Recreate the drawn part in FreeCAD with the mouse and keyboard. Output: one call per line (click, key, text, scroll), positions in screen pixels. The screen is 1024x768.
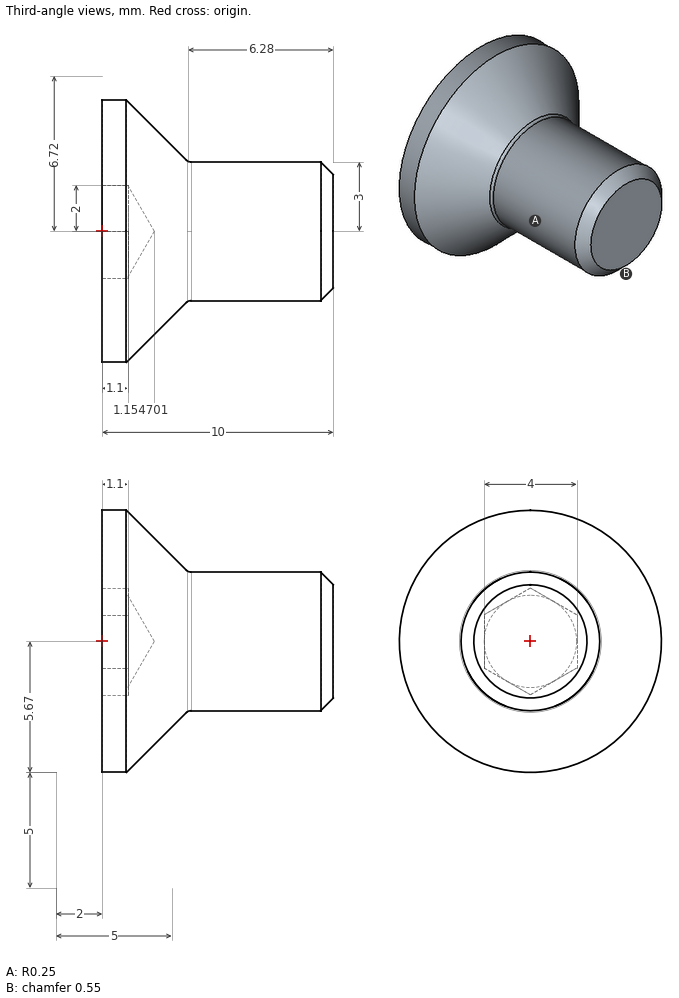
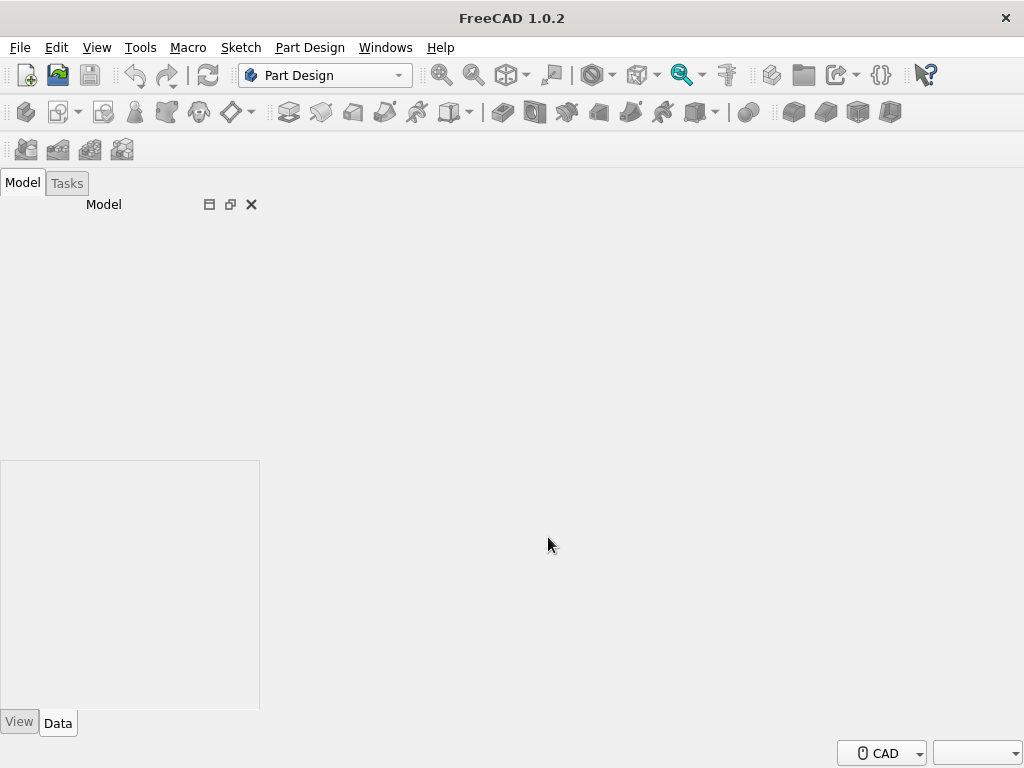
key(ctrl+n)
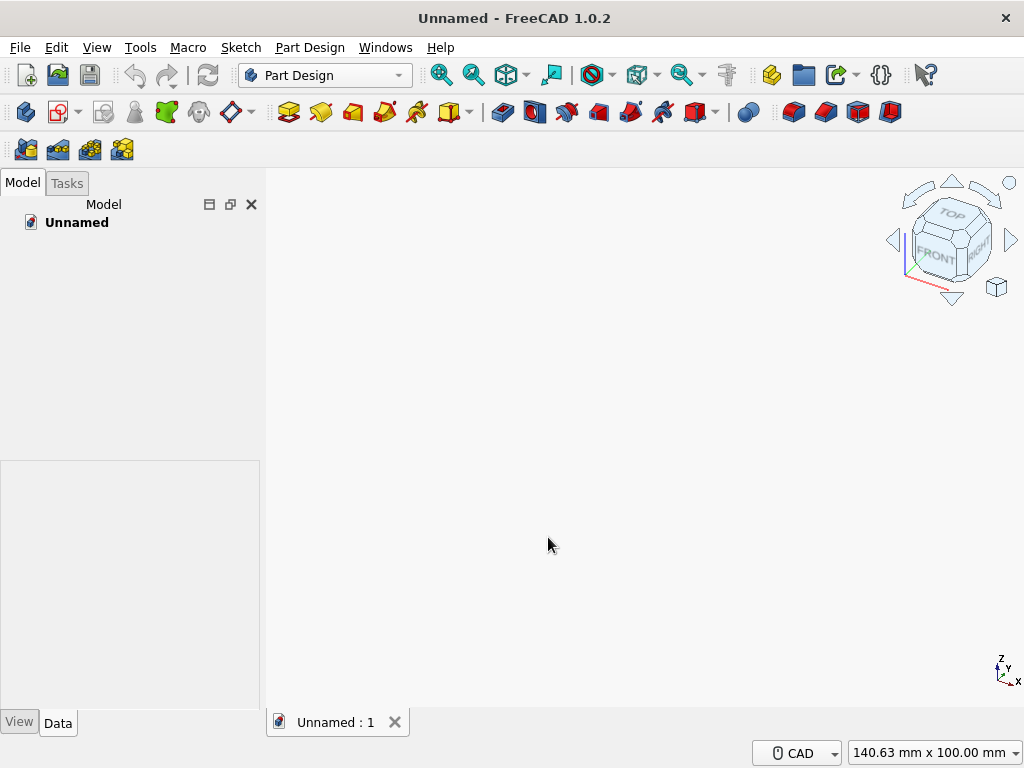
click(58, 112)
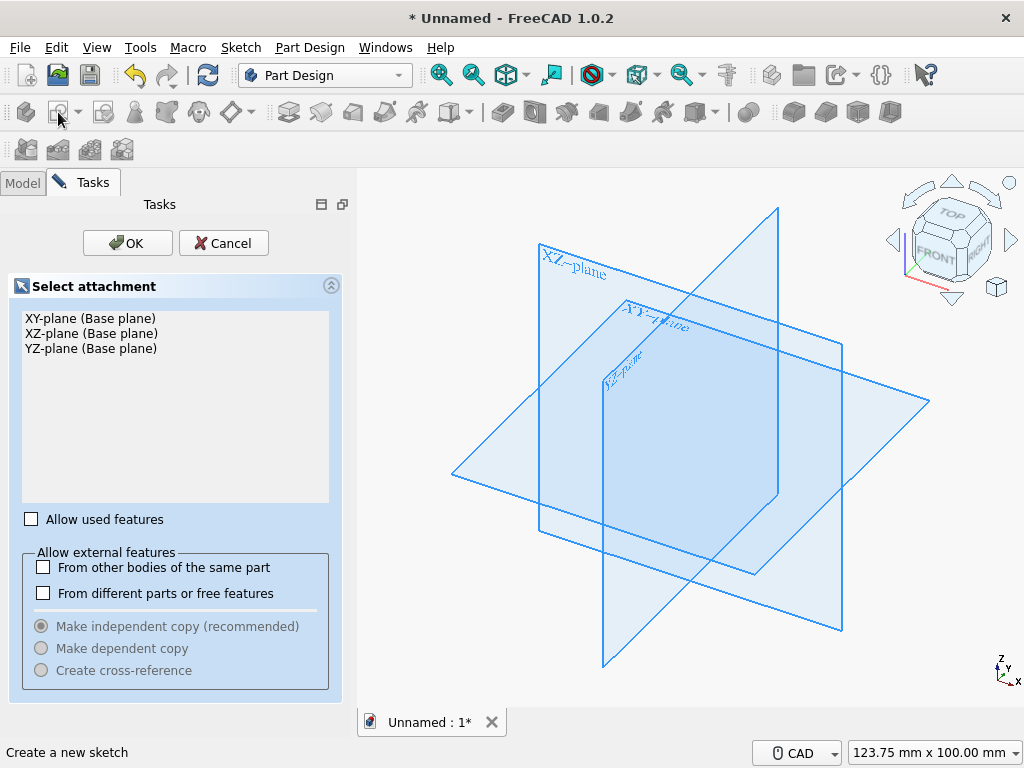
click(82, 318)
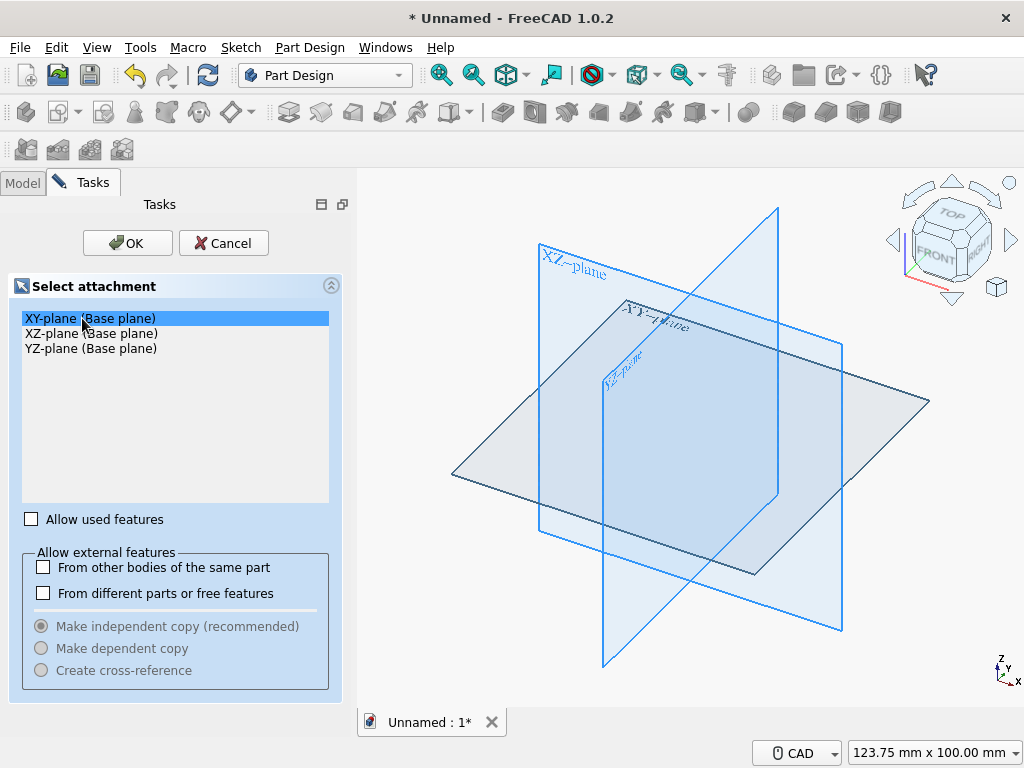
click(128, 243)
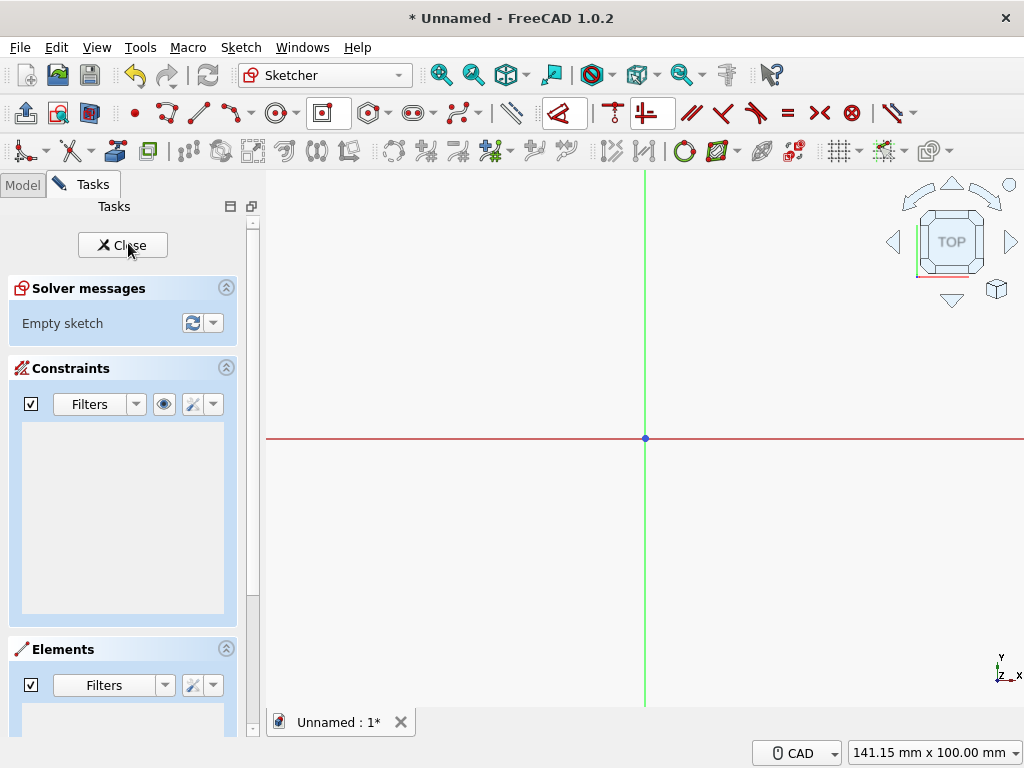
scroll(687, 418, up, 10)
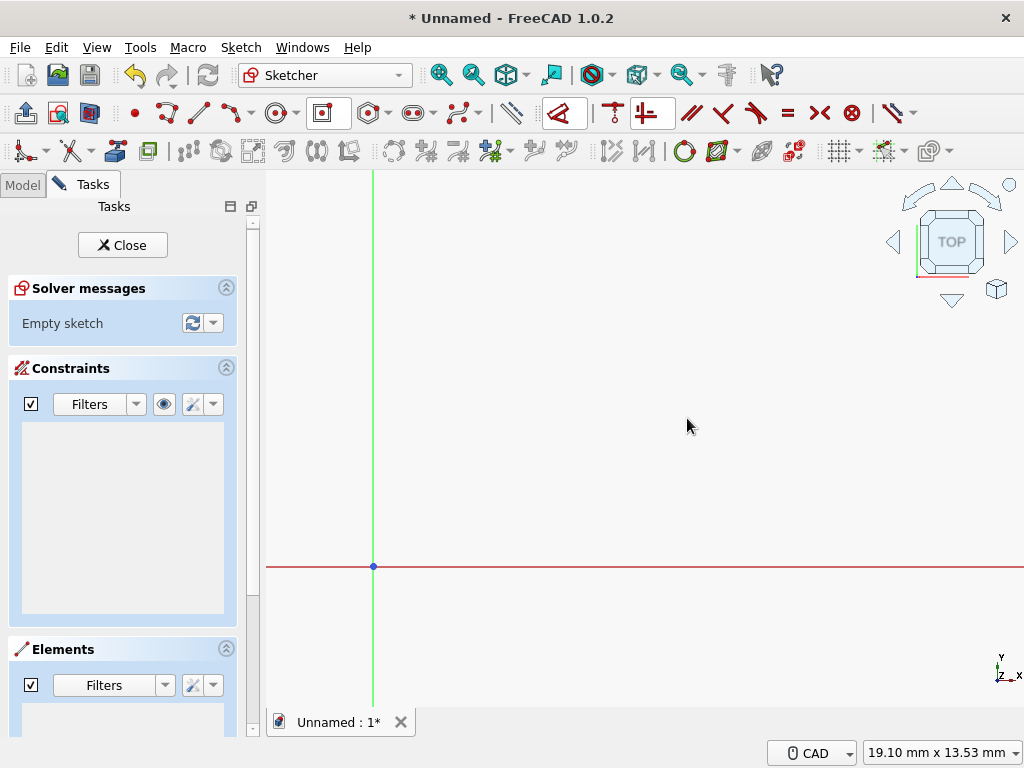
key(g)
key(m)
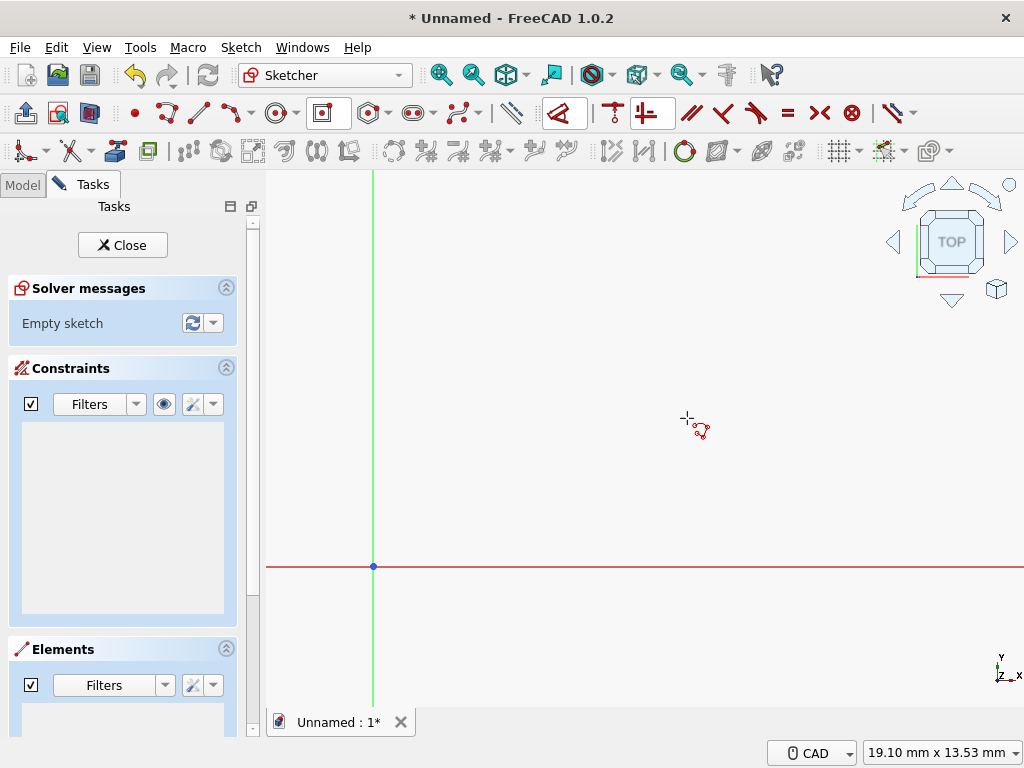
click(373, 567)
click(770, 558)
click(770, 447)
click(521, 447)
click(382, 300)
click(373, 567)
key(Escape)
key(Escape)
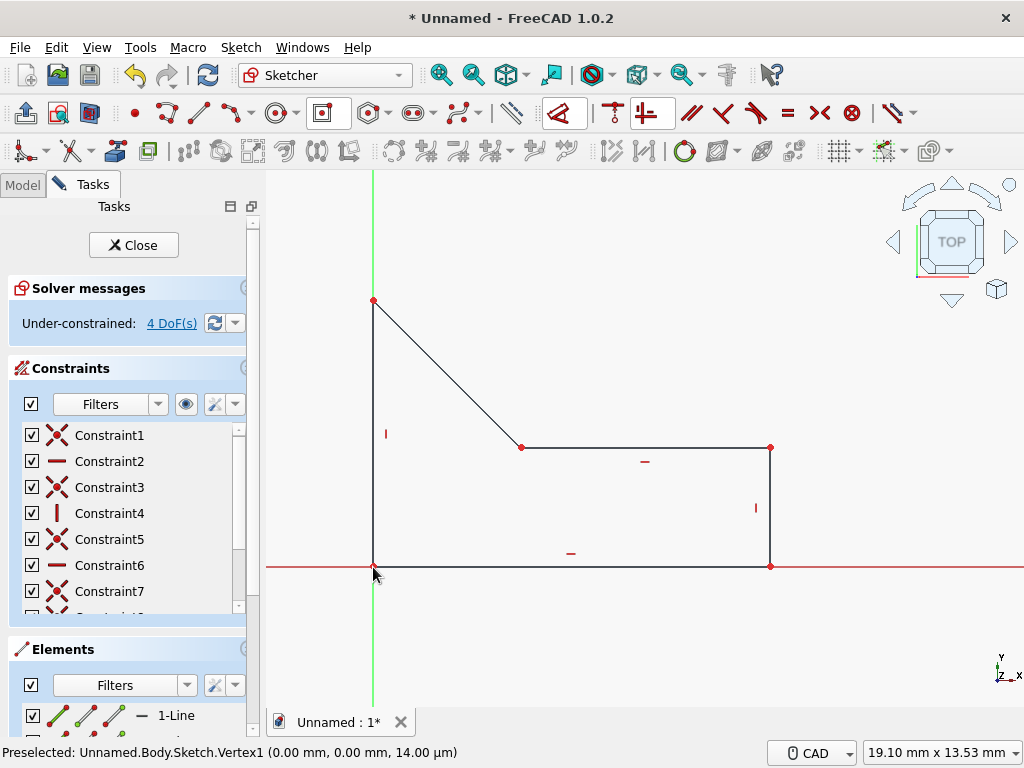
key(d)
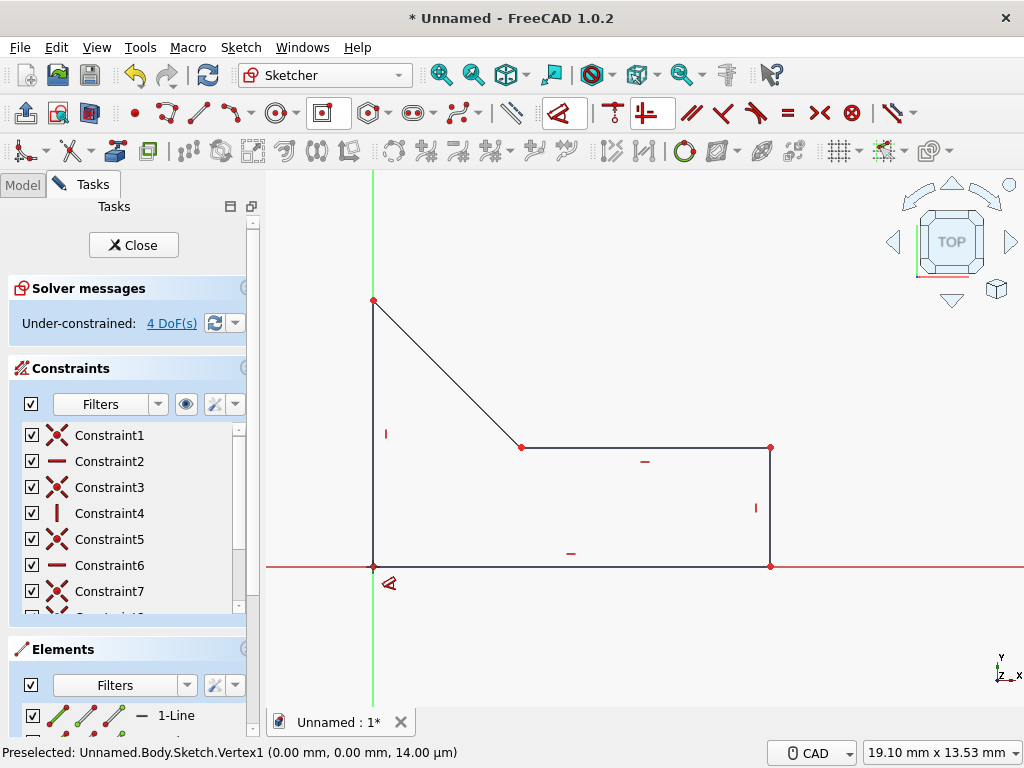
click(770, 531)
click(804, 507)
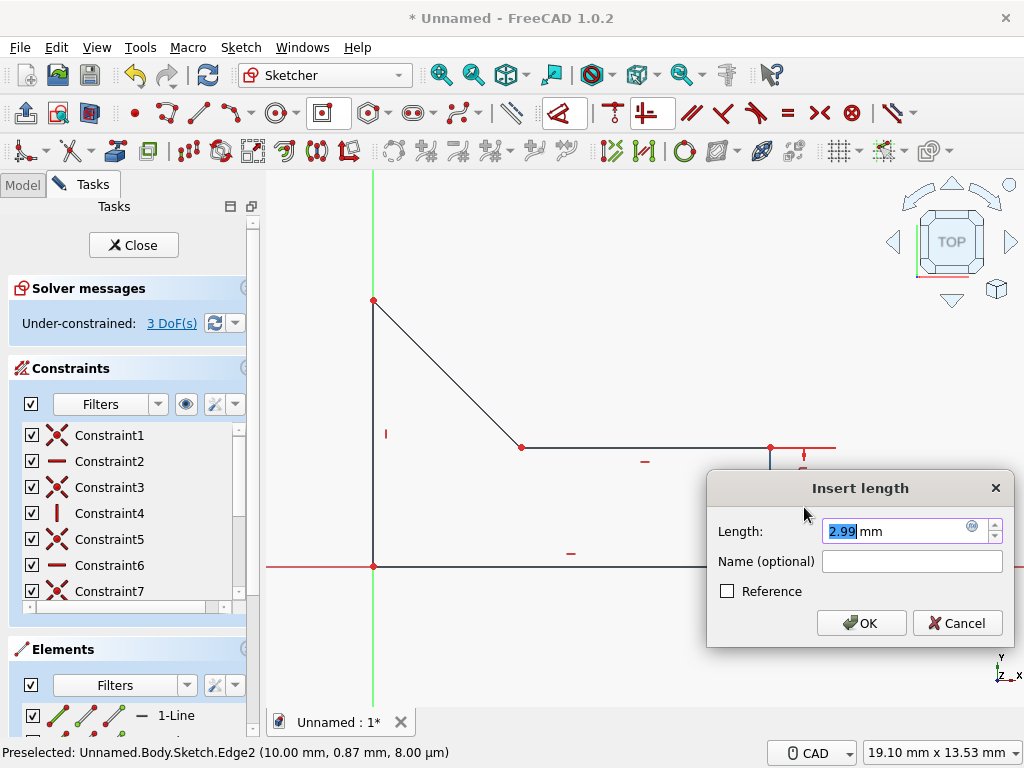
text(3)
key(Return)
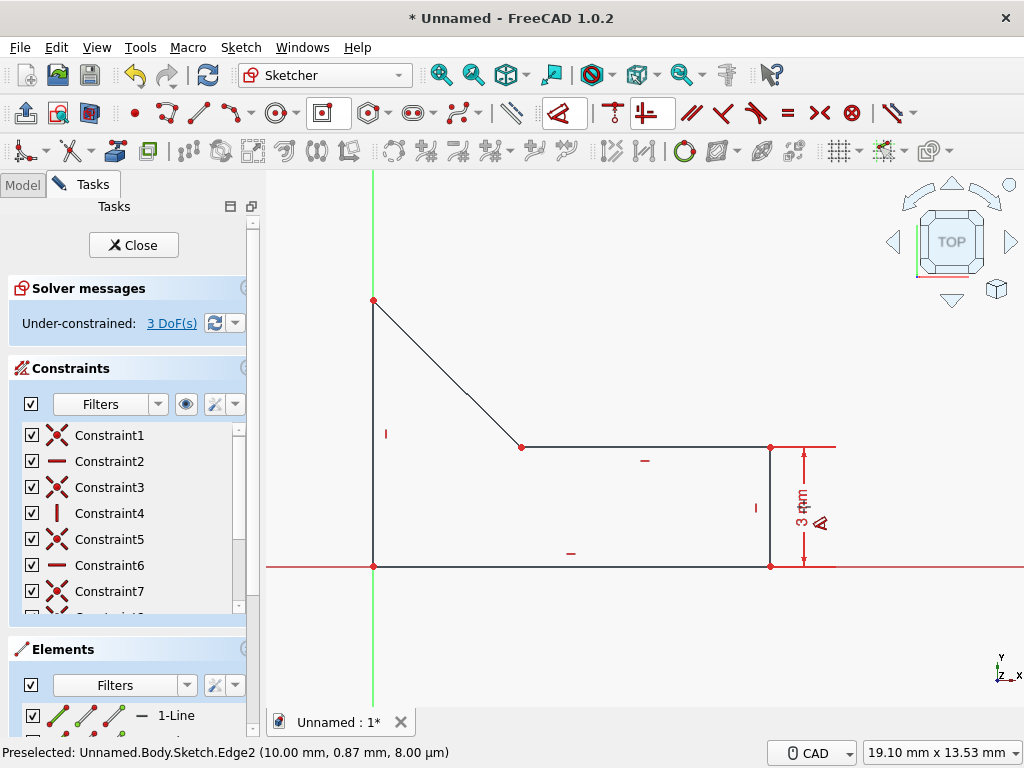
click(492, 567)
click(572, 601)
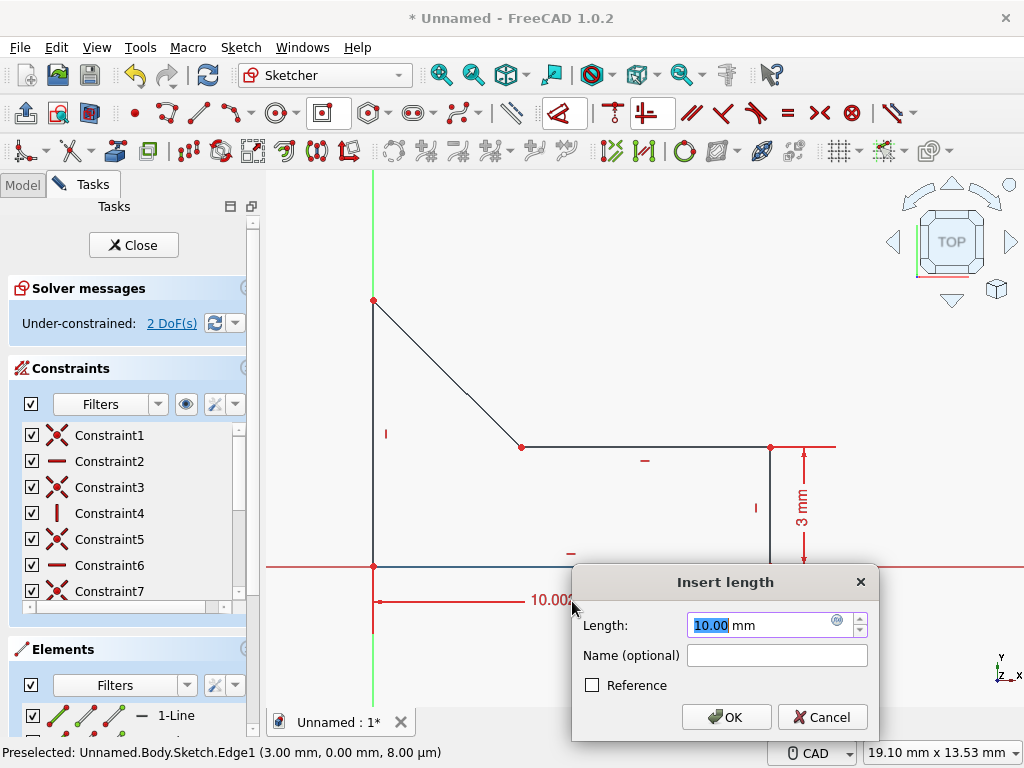
text(10)
key(Return)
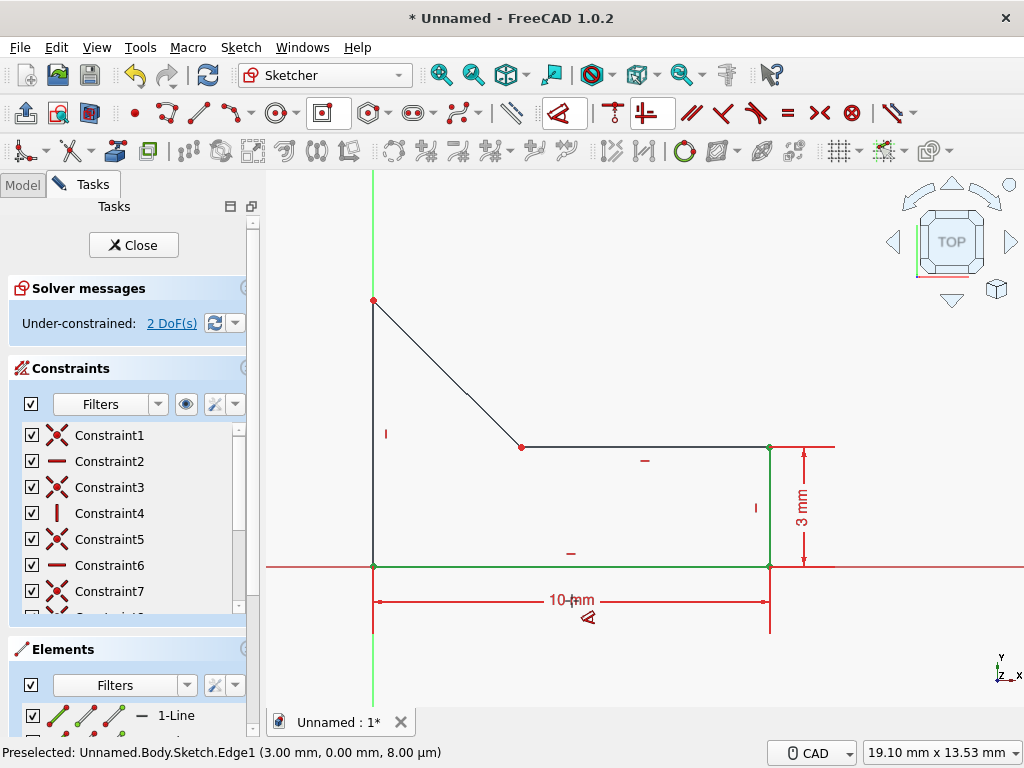
click(695, 447)
click(645, 481)